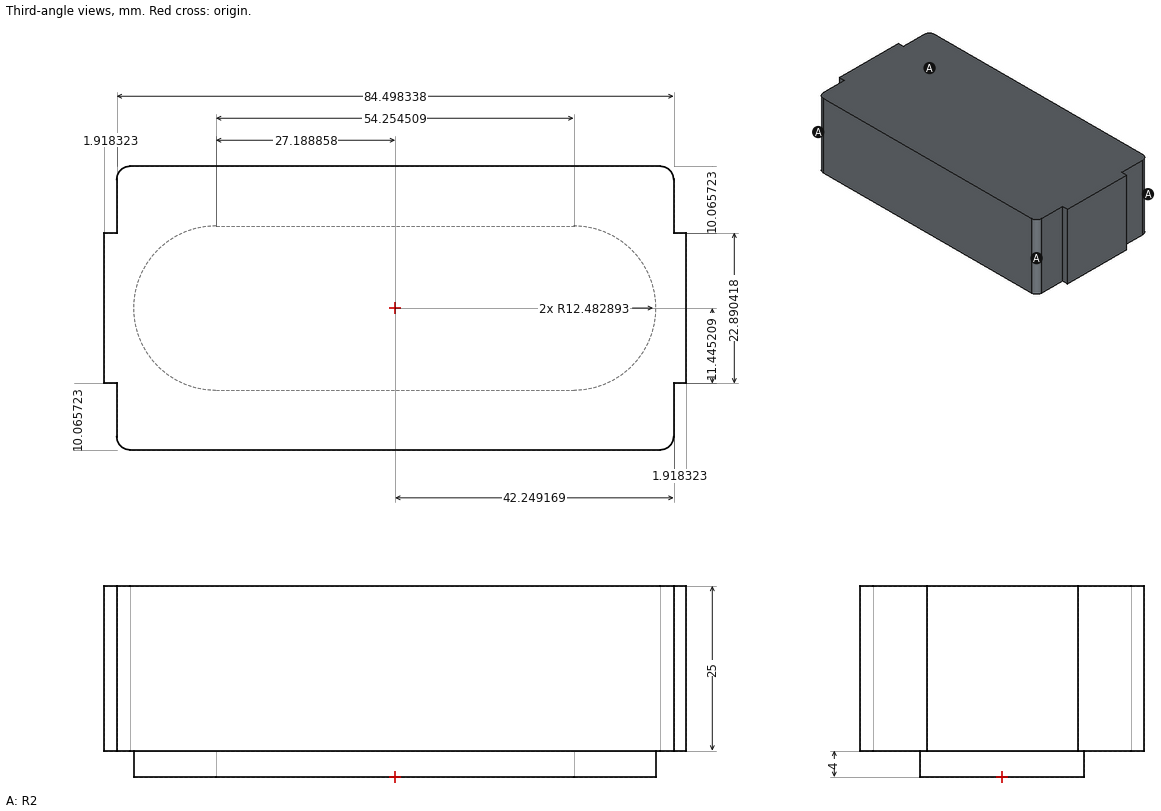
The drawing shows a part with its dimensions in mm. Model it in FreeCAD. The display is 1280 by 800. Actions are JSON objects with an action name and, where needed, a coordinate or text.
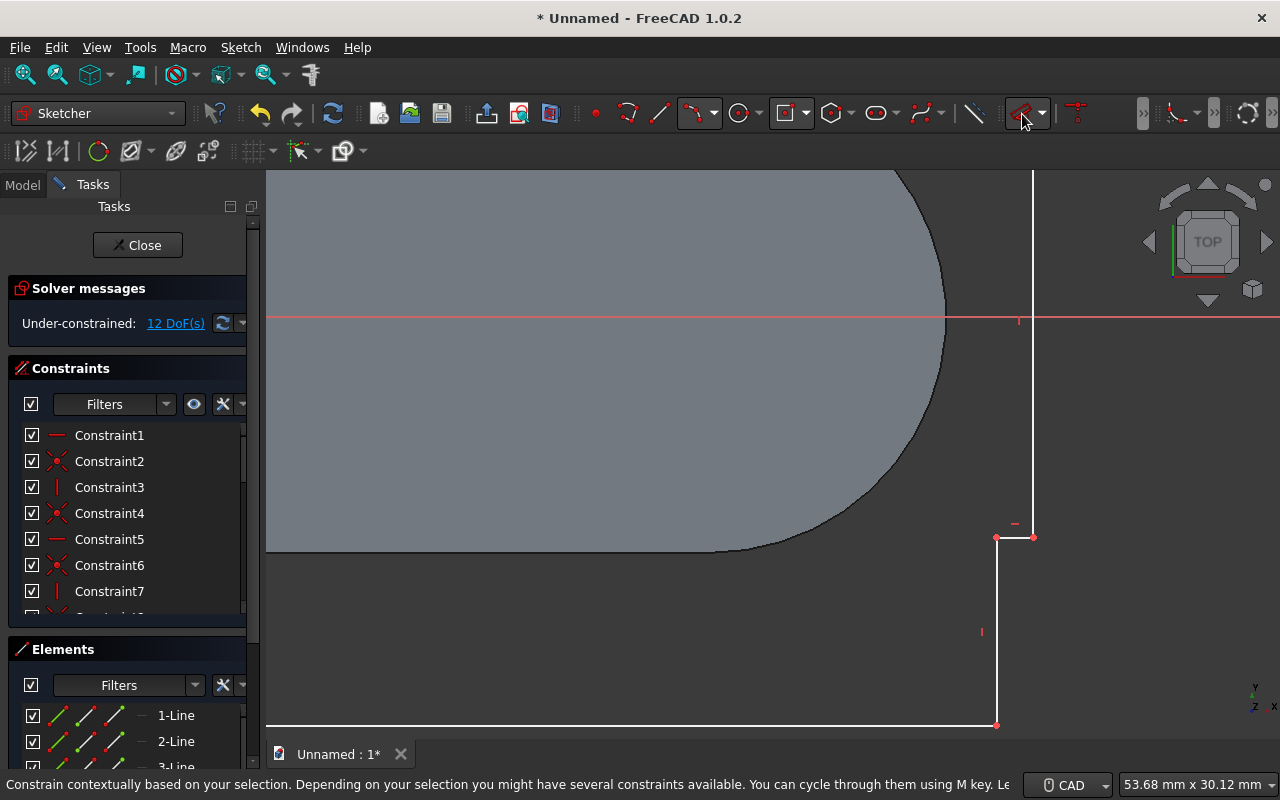
{"action": "scroll", "coordinate": [1008, 538], "scroll_direction": "up", "scroll_amount": 2}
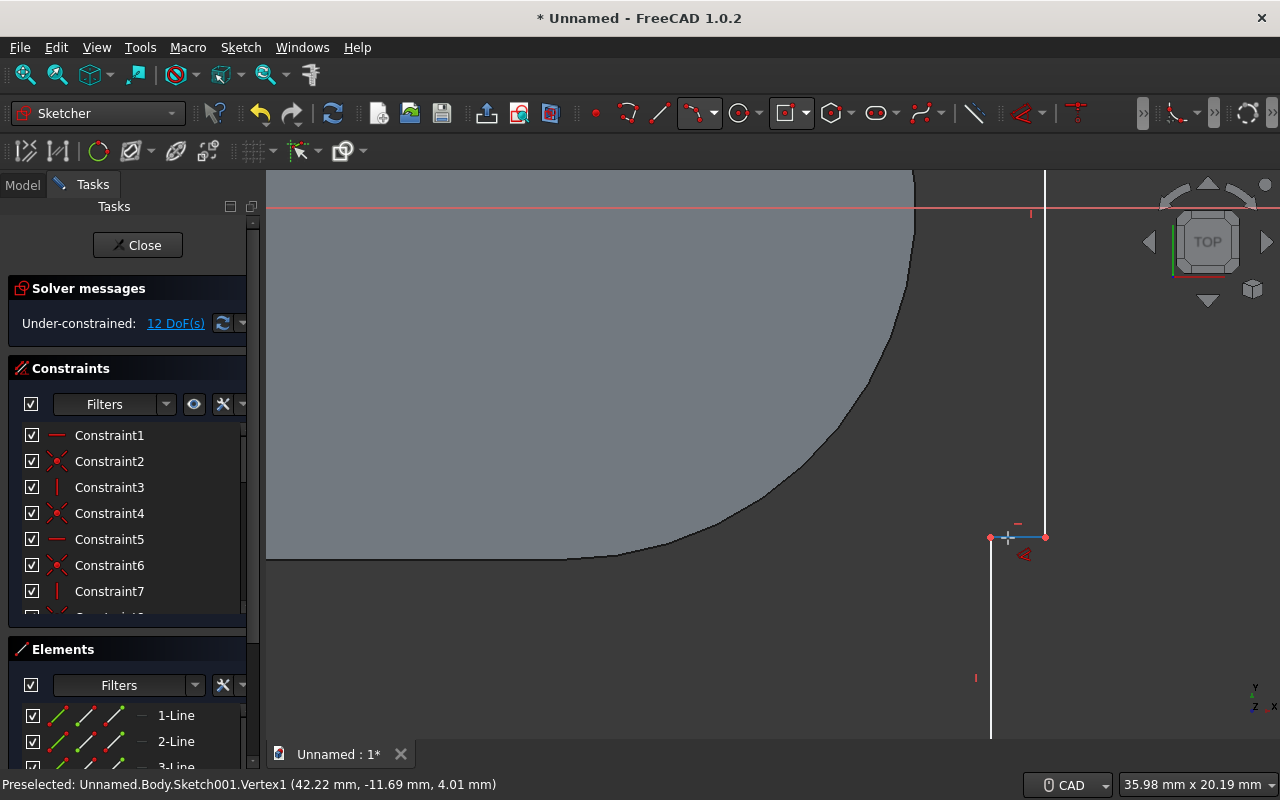
{"action": "left_click", "coordinate": [1007, 537]}
{"action": "left_click", "coordinate": [1018, 571]}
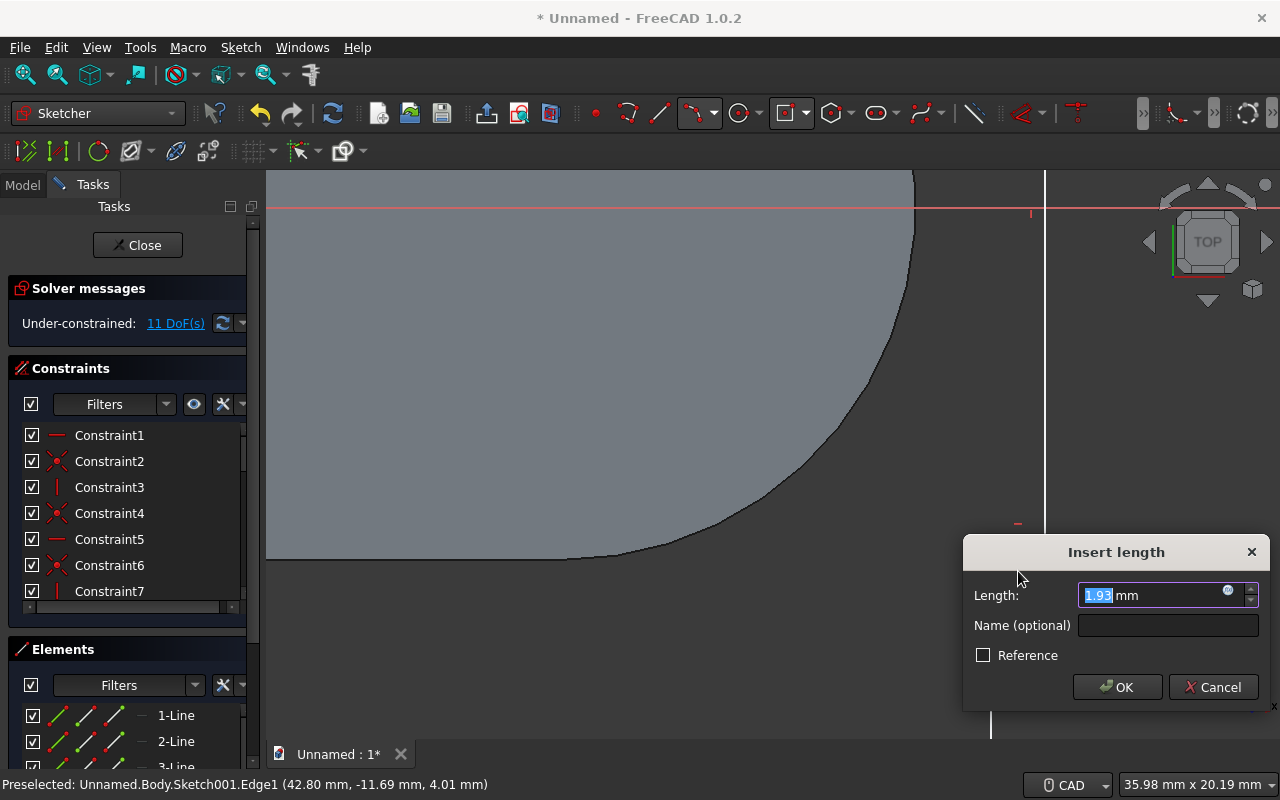
{"action": "type", "text": "1.918323"}
{"action": "key", "text": "Return"}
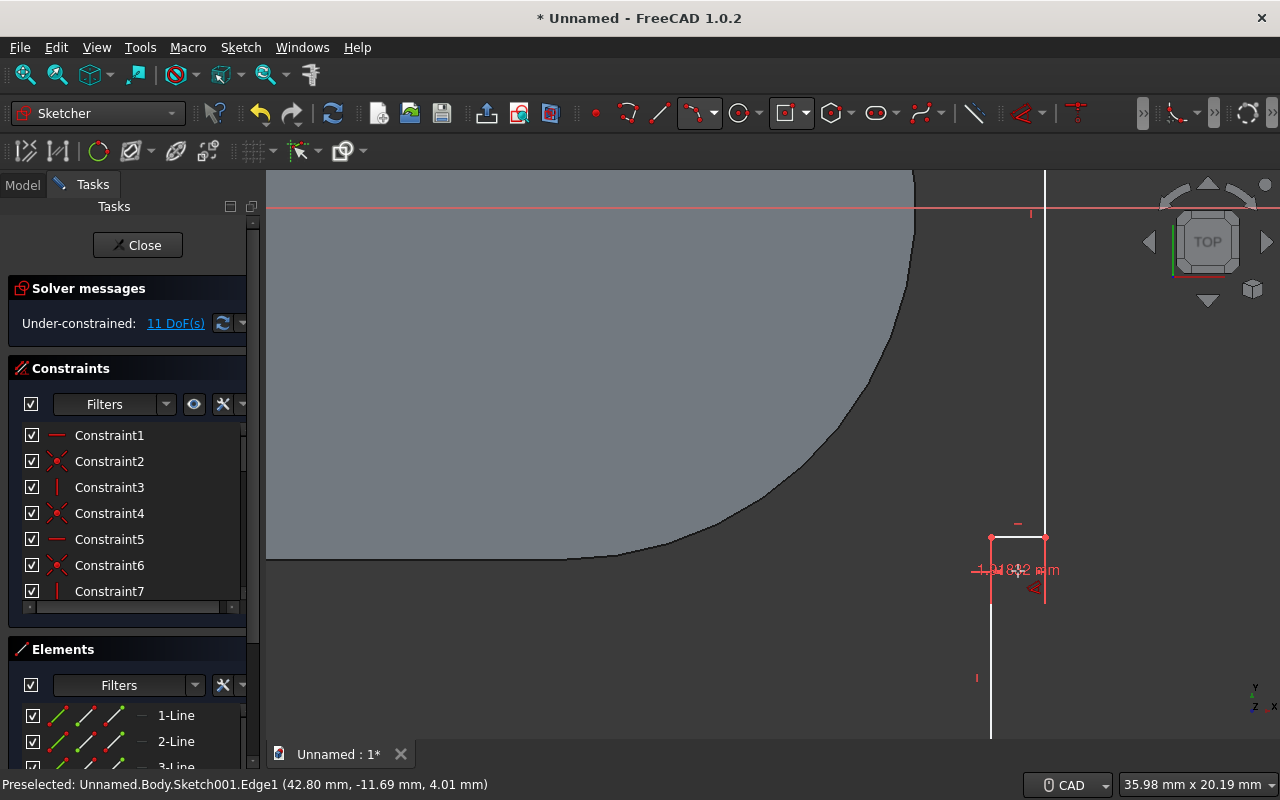
{"action": "scroll", "coordinate": [1000, 535], "scroll_direction": "down", "scroll_amount": 7}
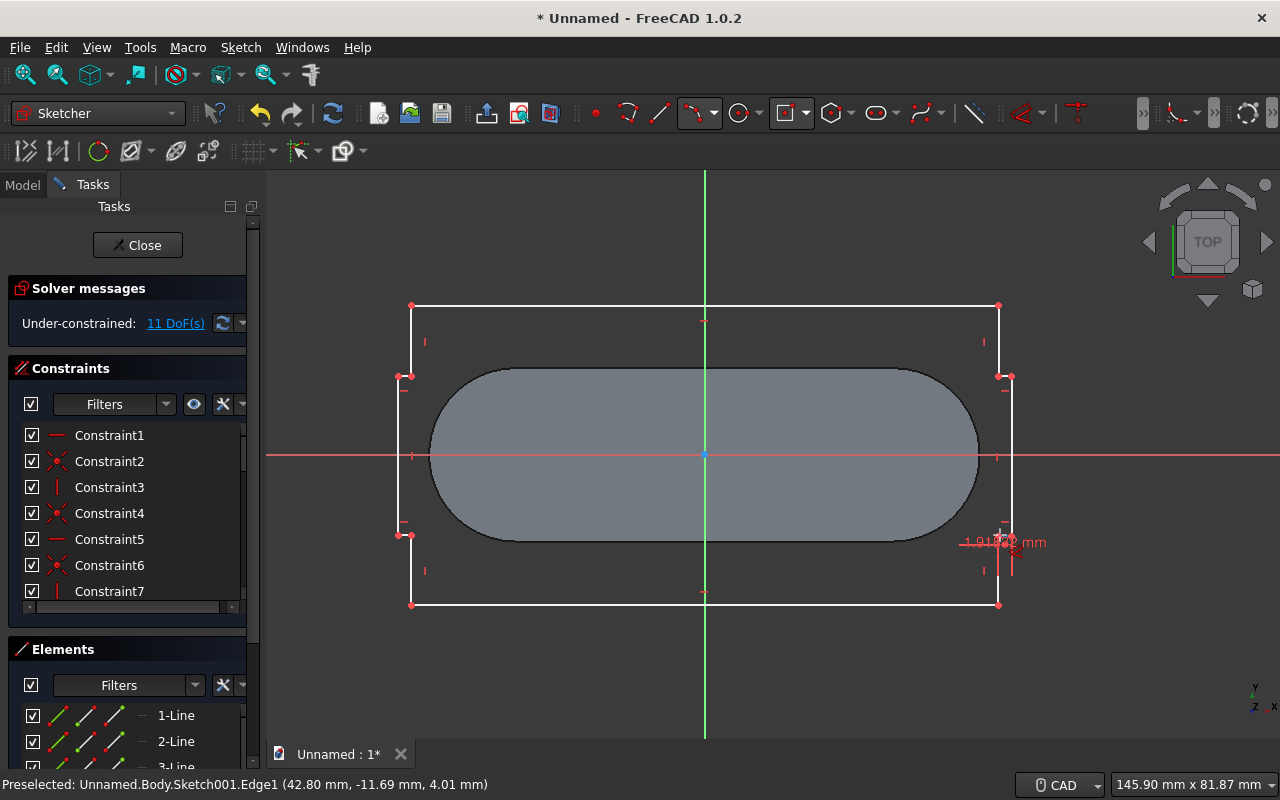
{"action": "scroll", "coordinate": [1008, 376], "scroll_direction": "up", "scroll_amount": 7}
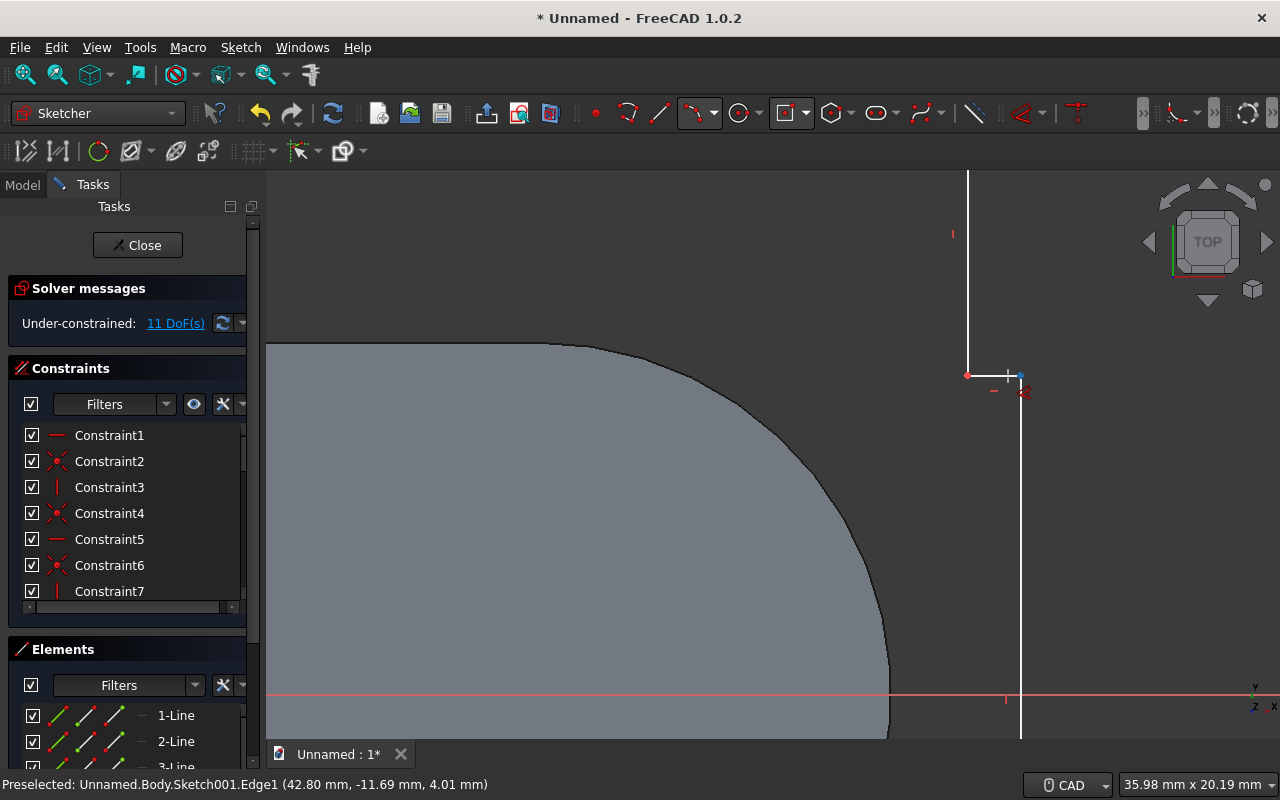
{"action": "left_click", "coordinate": [1005, 376]}
{"action": "left_click", "coordinate": [994, 342]}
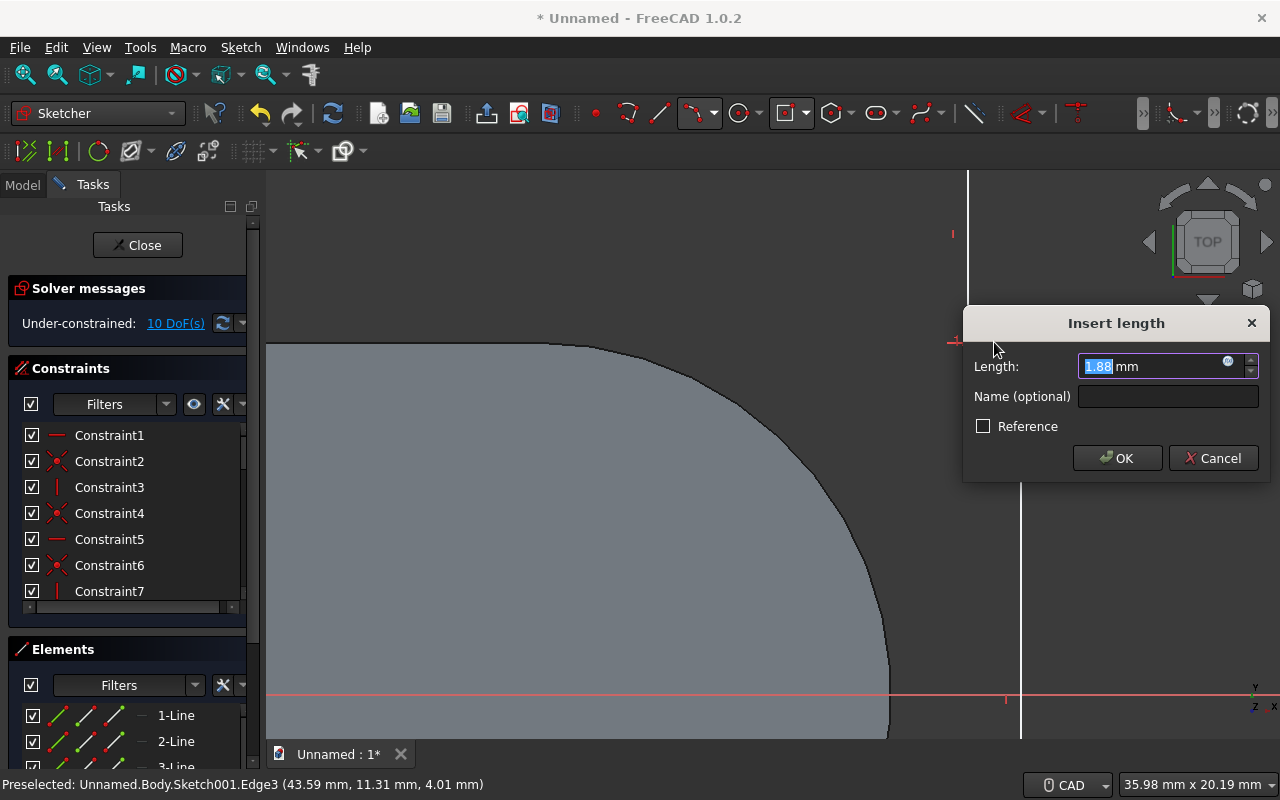
{"action": "type", "text": "1.918323"}
{"action": "key", "text": "Return"}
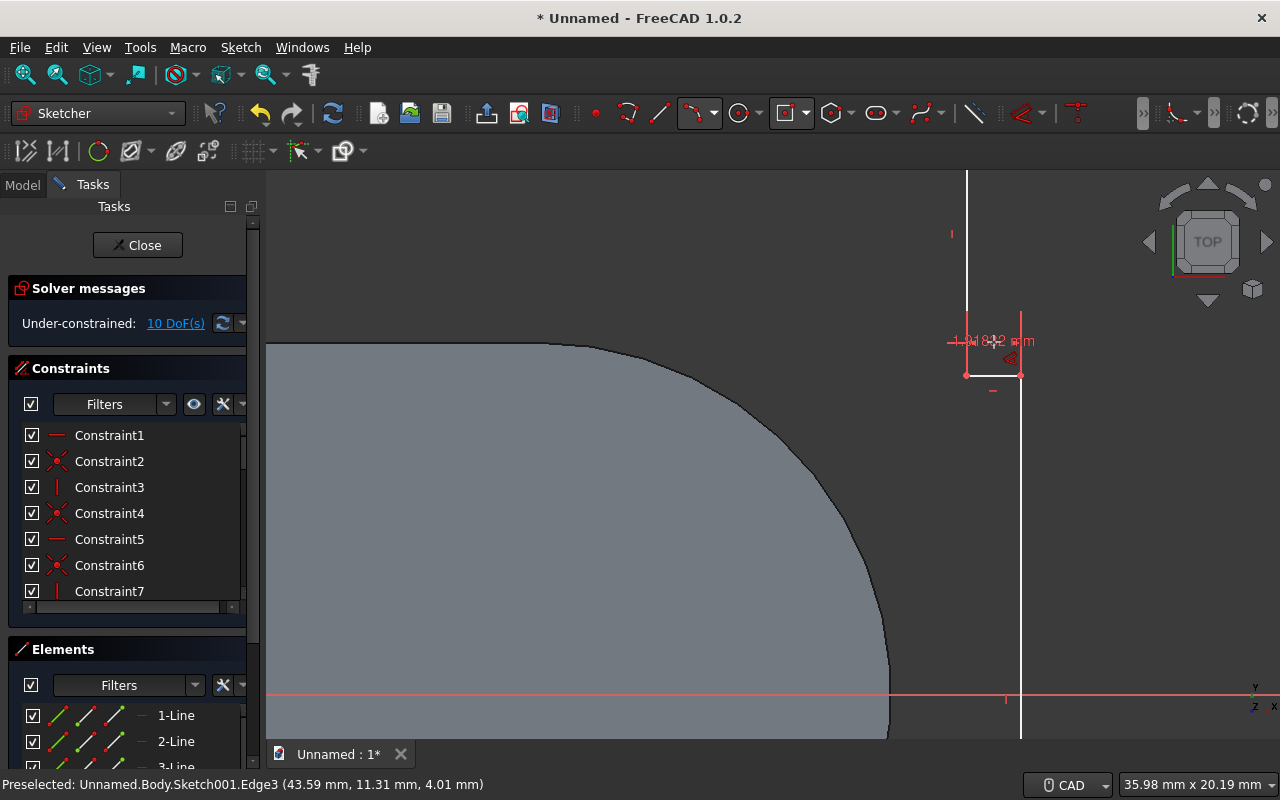
{"action": "scroll", "coordinate": [1008, 376], "scroll_direction": "down", "scroll_amount": 7}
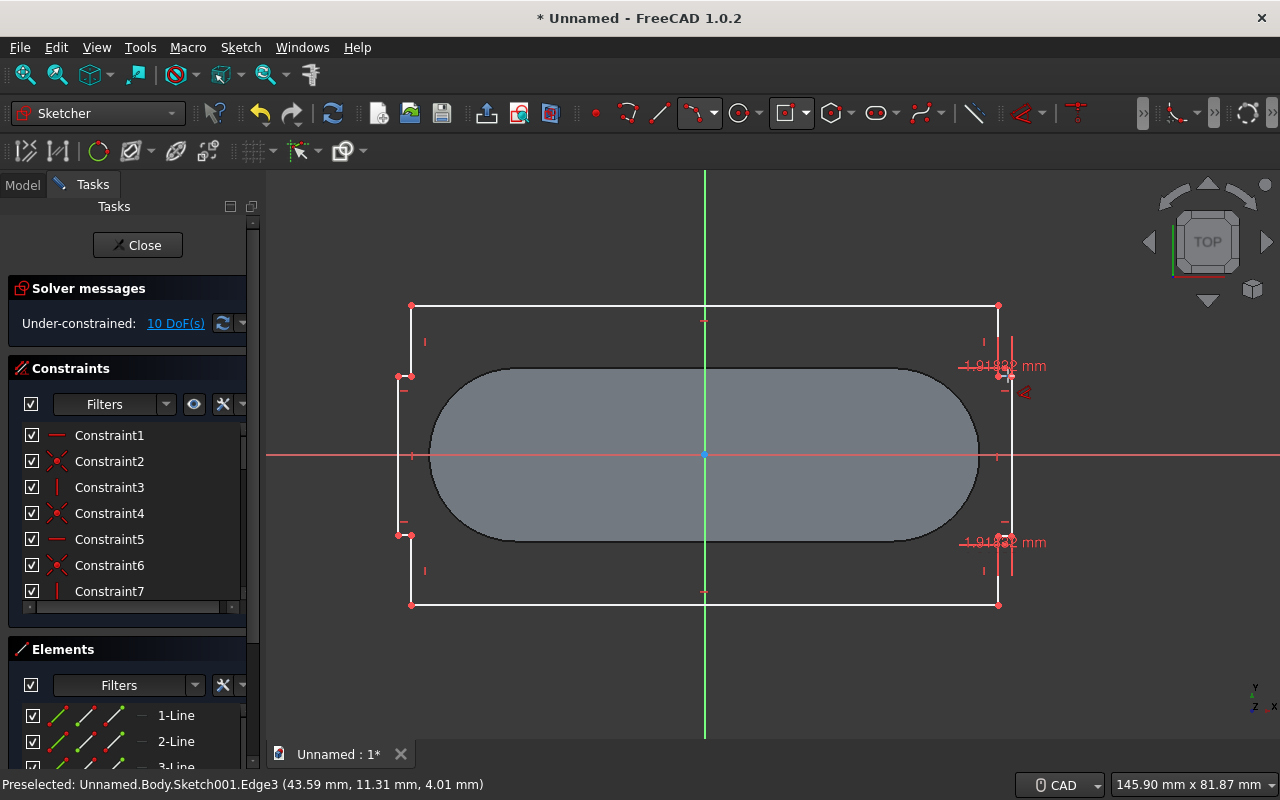
{"action": "scroll", "coordinate": [407, 376], "scroll_direction": "up", "scroll_amount": 7}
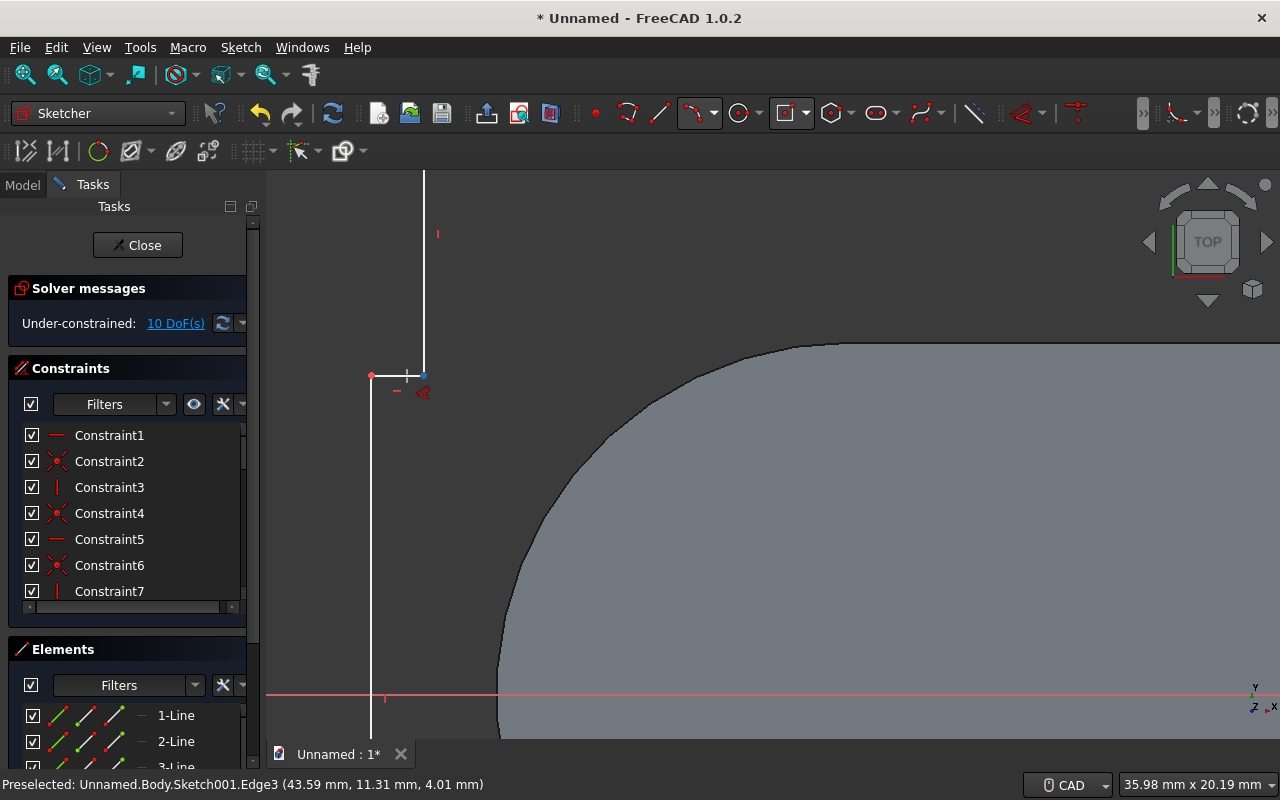
{"action": "left_click", "coordinate": [408, 376]}
{"action": "left_click", "coordinate": [398, 342]}